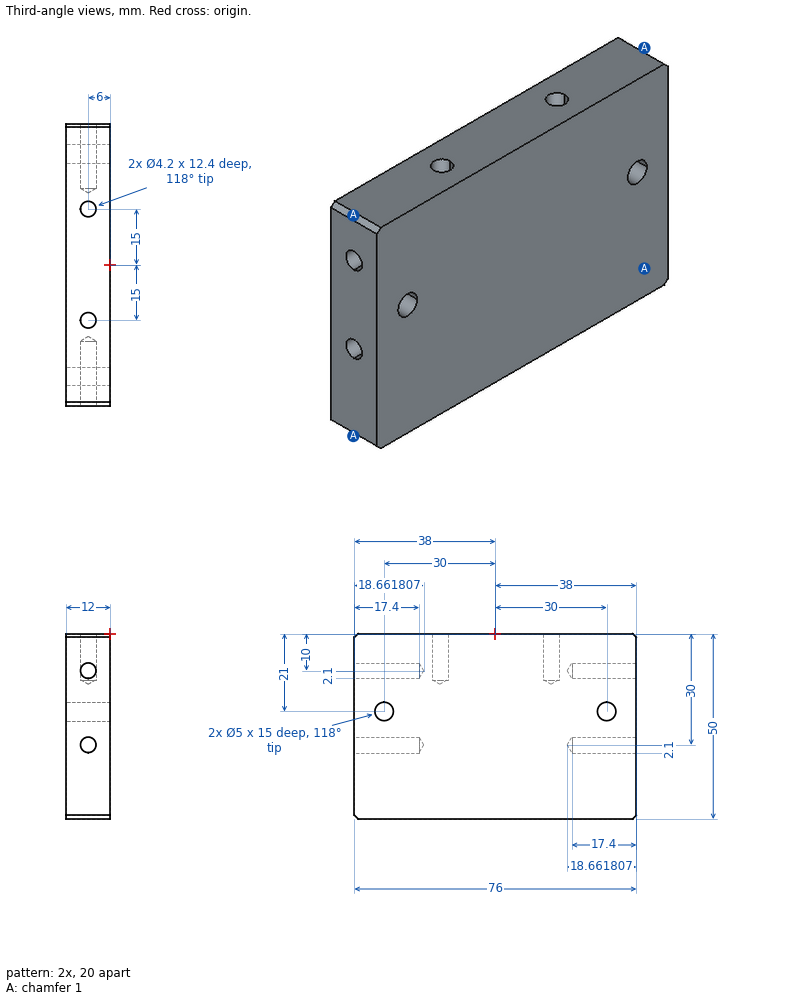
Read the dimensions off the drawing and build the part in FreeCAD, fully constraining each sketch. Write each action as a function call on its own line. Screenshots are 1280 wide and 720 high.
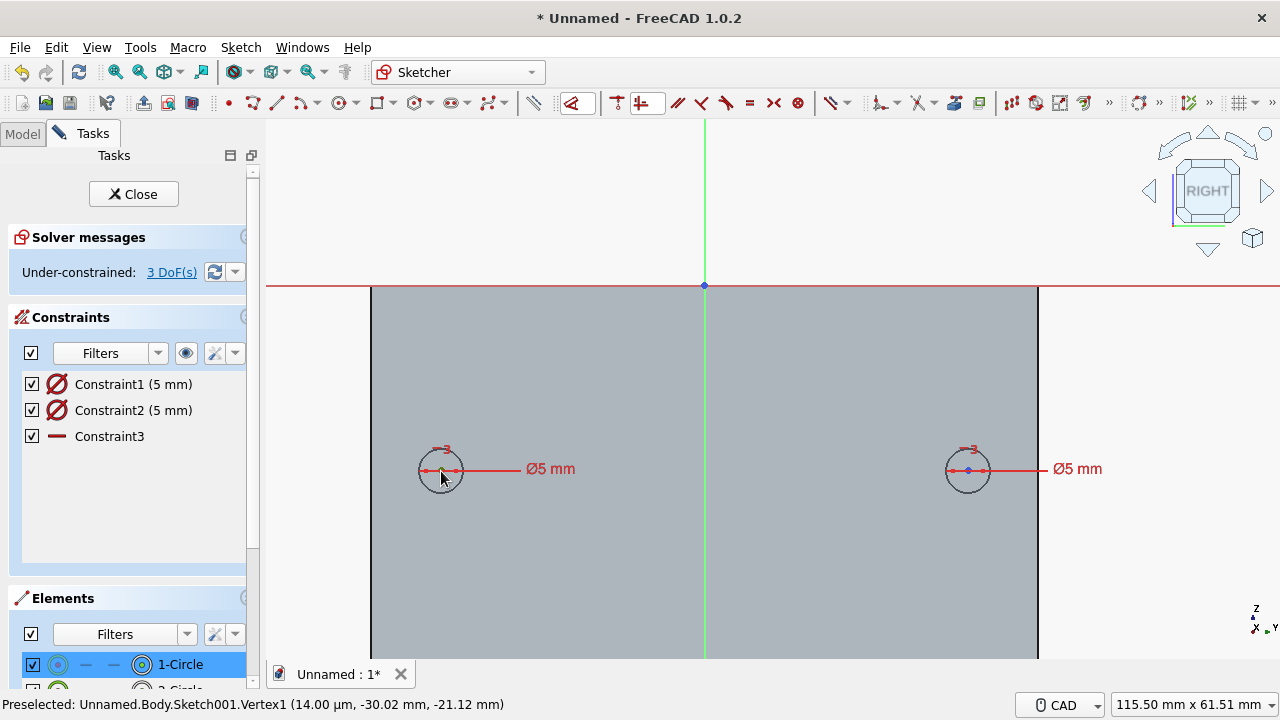
click(590, 104)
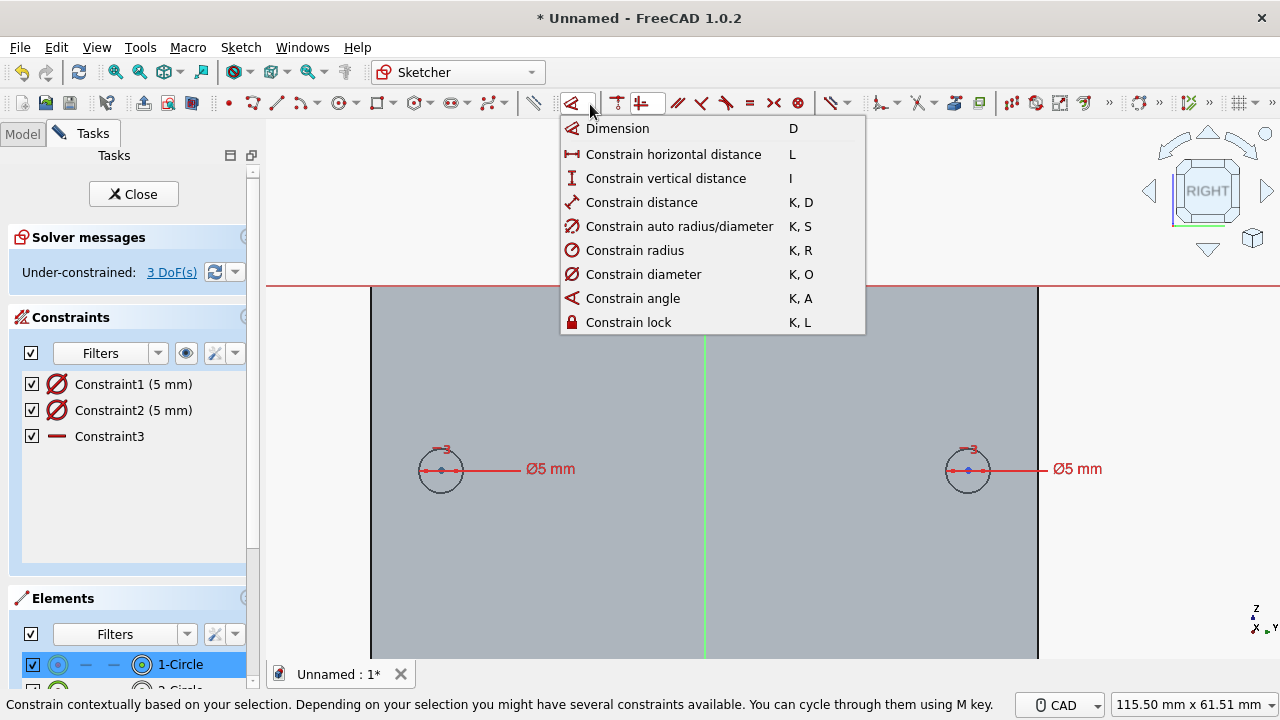
click(713, 154)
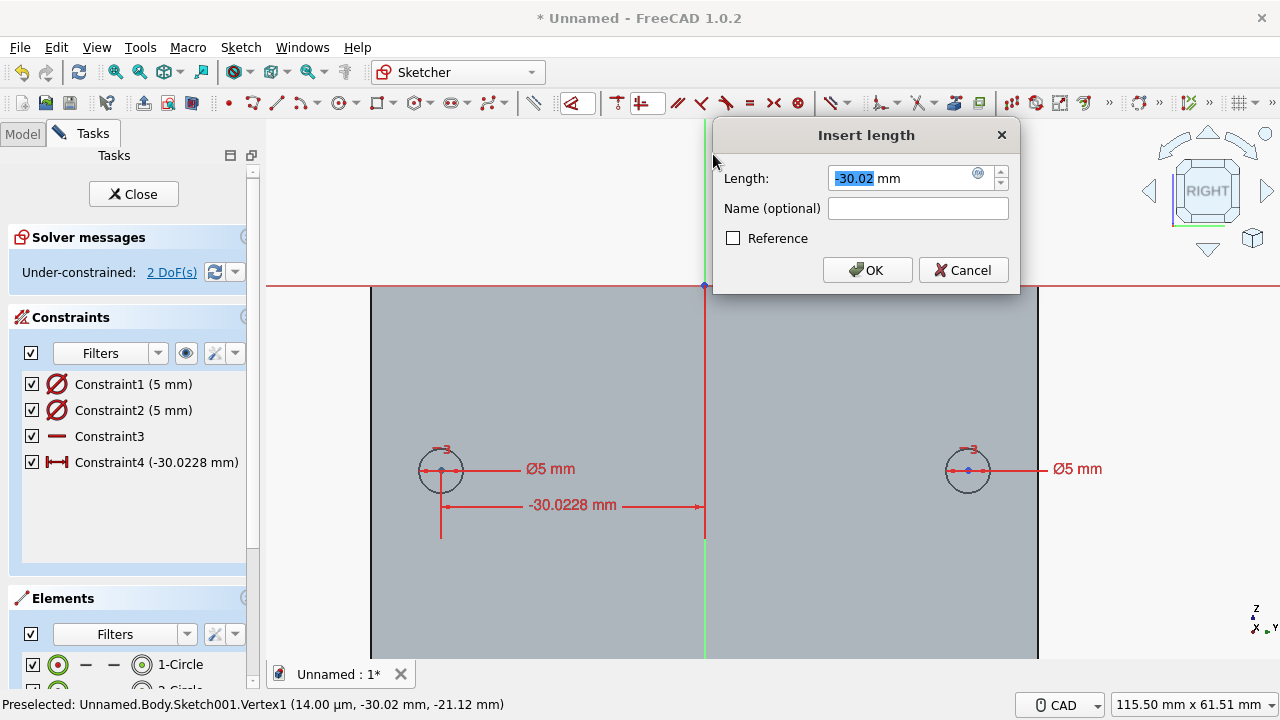
text(-30)
key(Return)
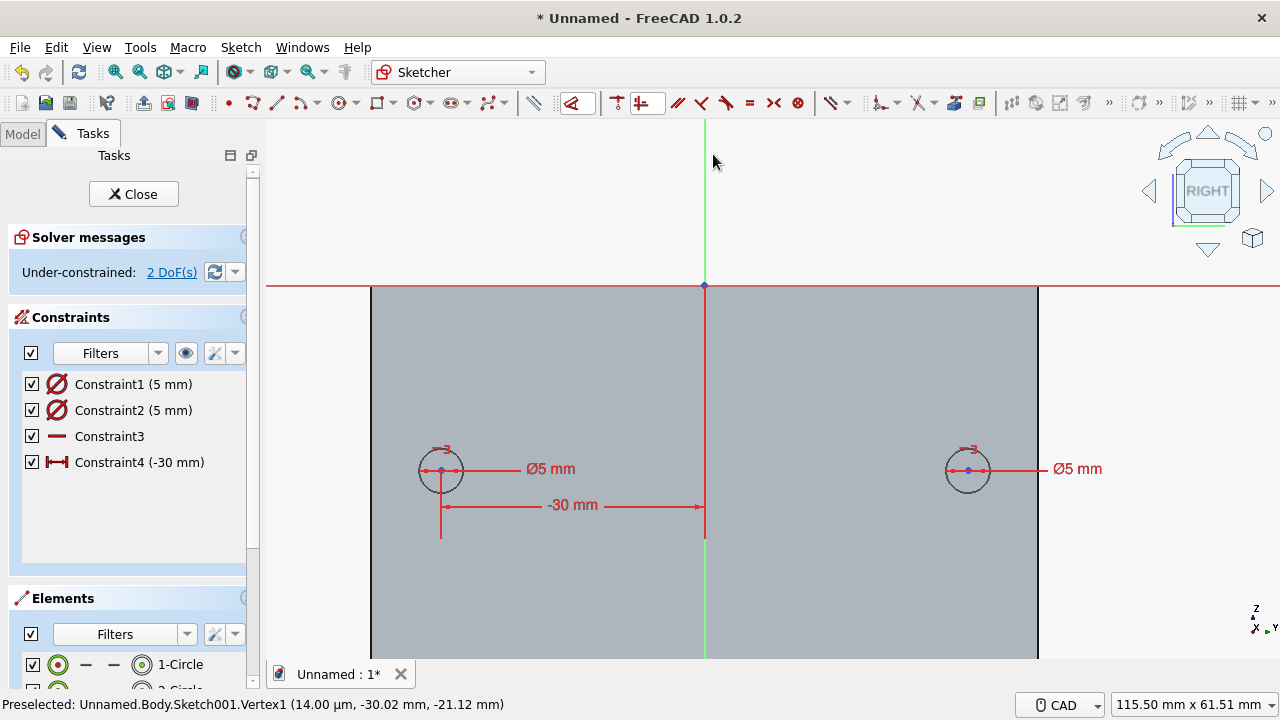
click(441, 471)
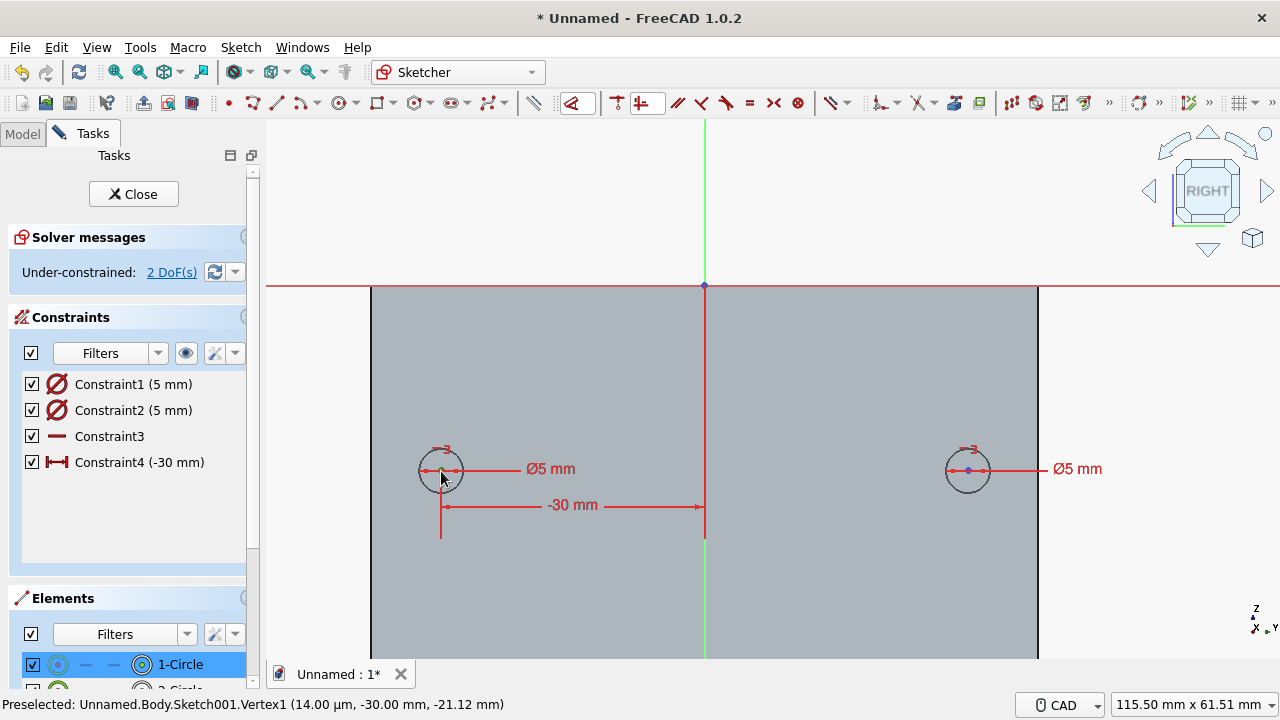
key(i)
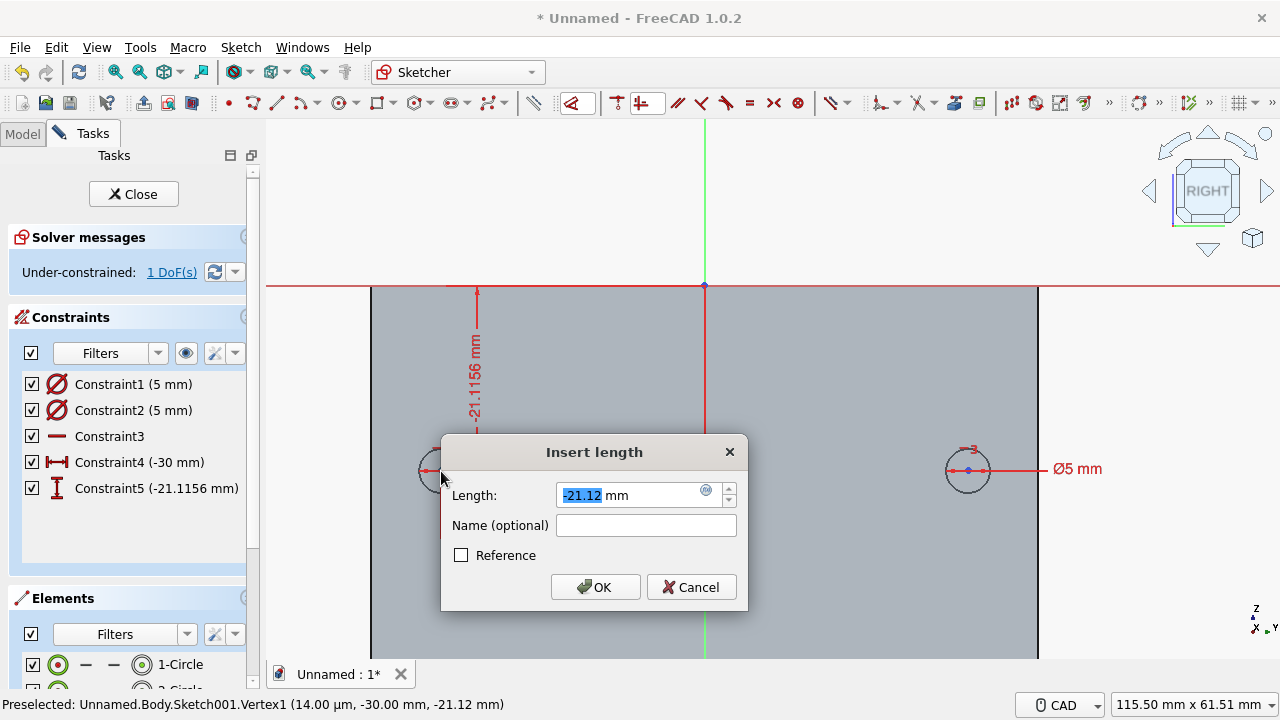
text(-21)
key(Return)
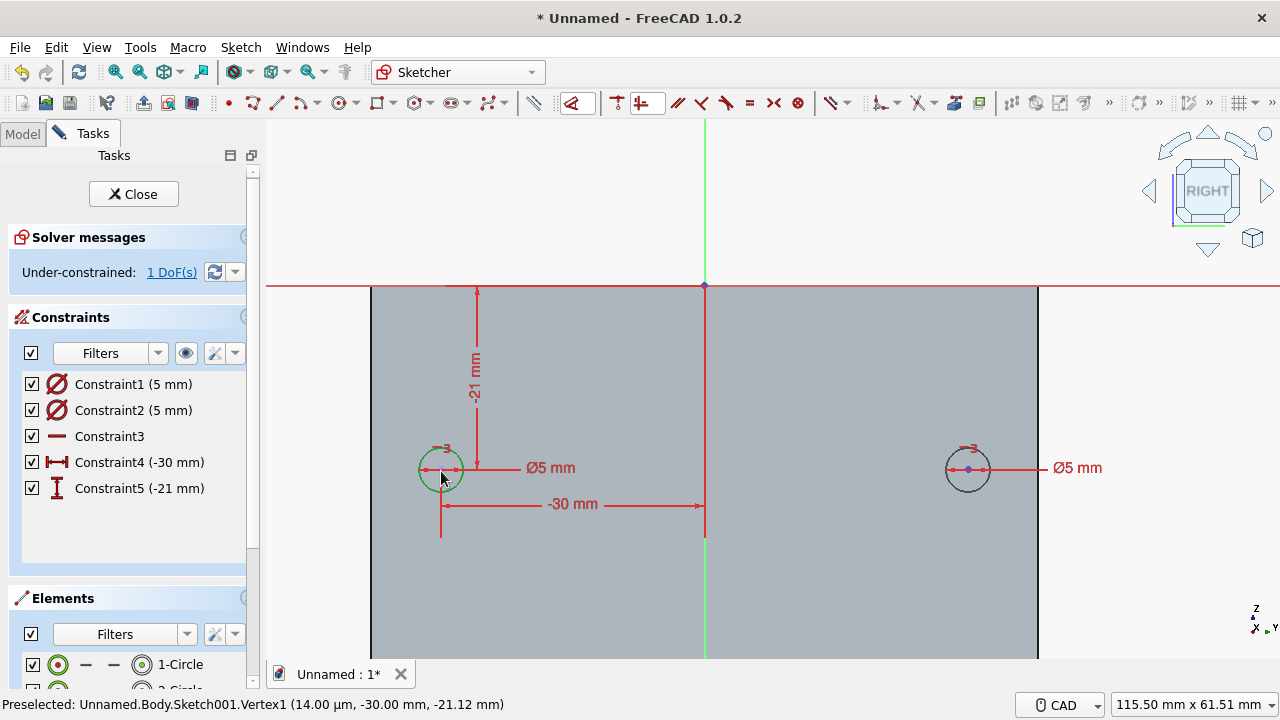
click(968, 470)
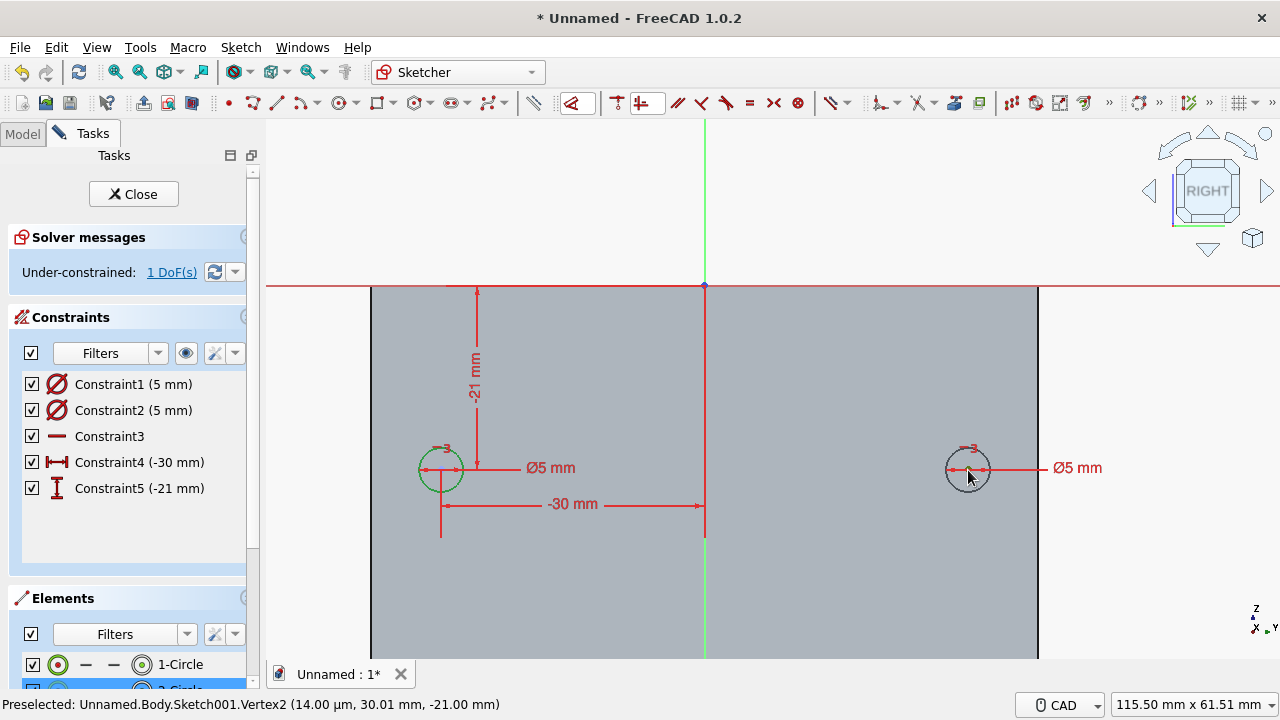
click(590, 104)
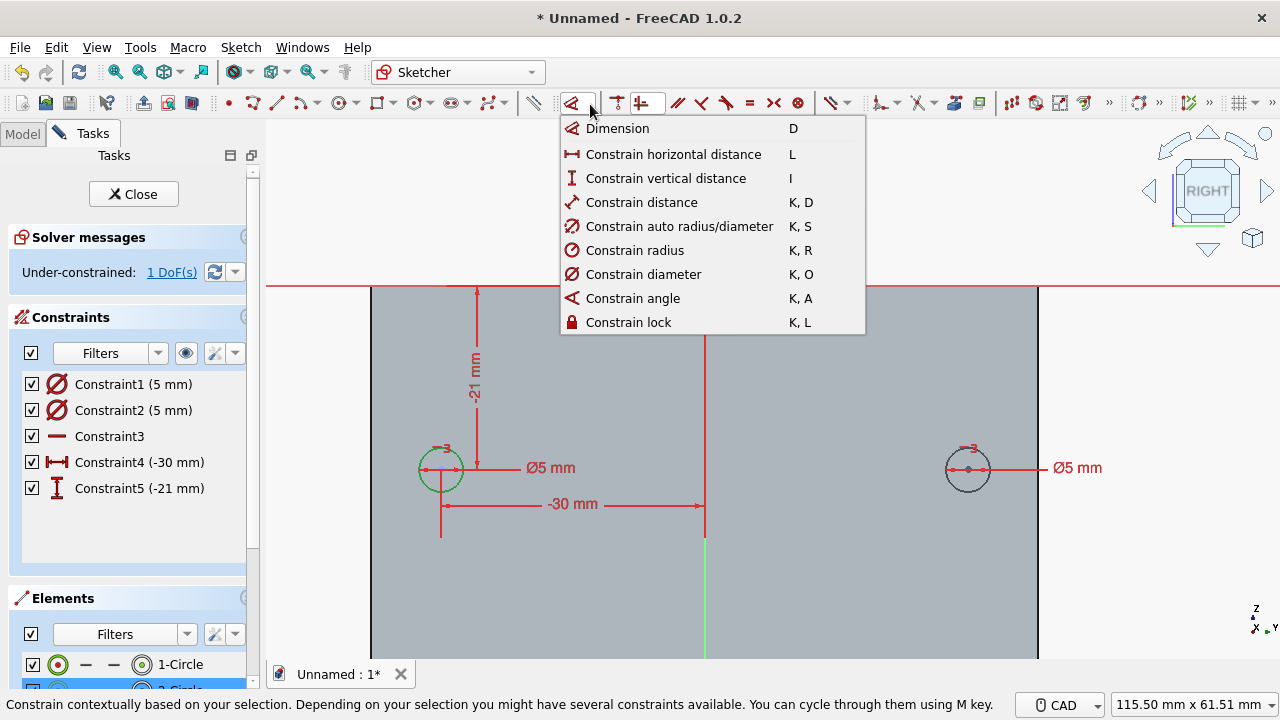
click(713, 154)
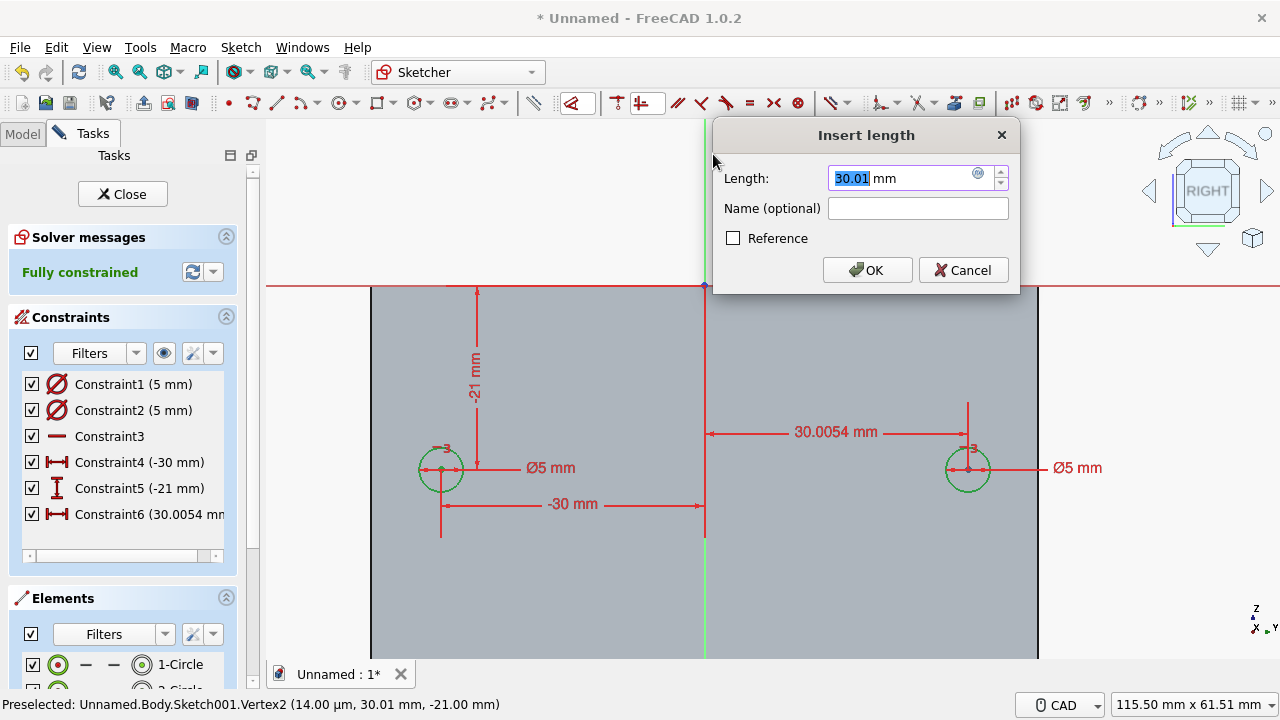
text(30)
key(Return)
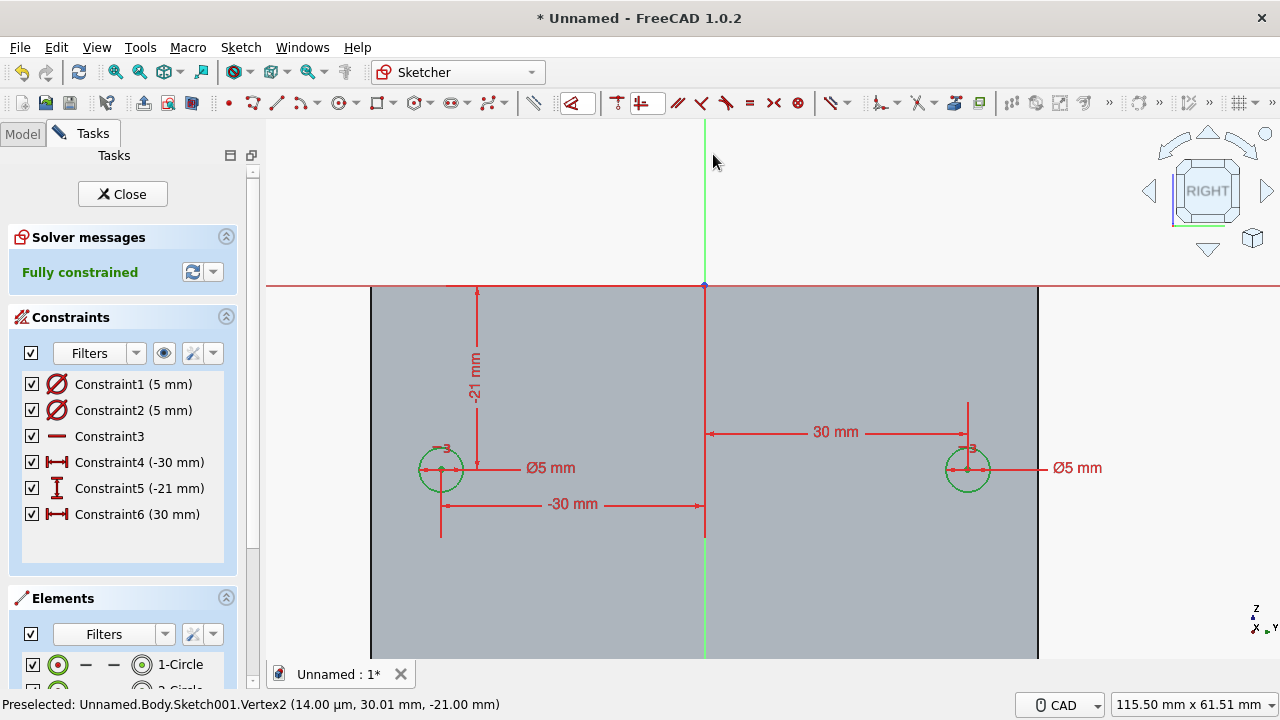
click(123, 194)